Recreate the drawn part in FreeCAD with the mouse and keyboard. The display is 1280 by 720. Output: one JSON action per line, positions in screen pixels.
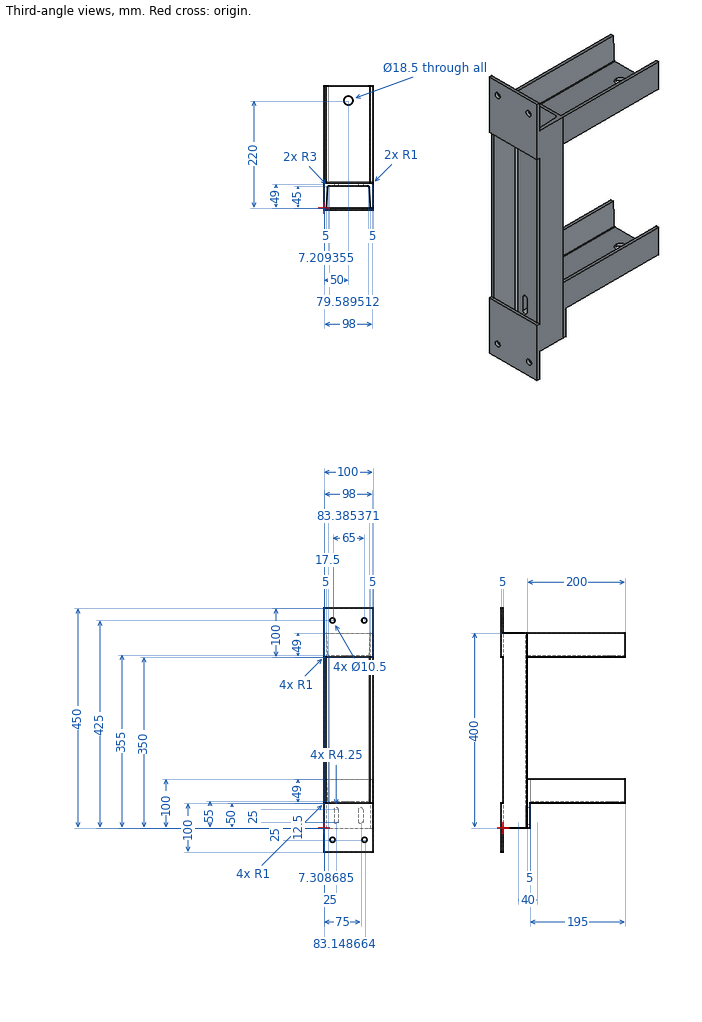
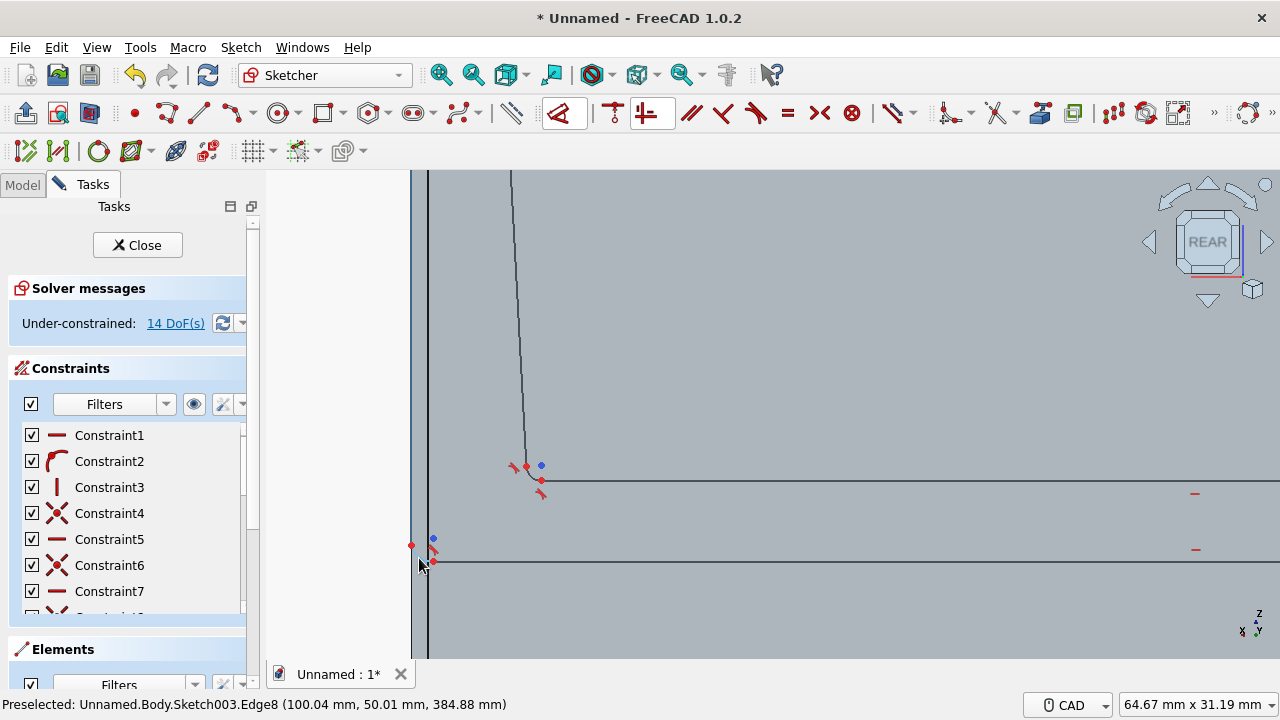
{"action": "left_click", "coordinate": [420, 557]}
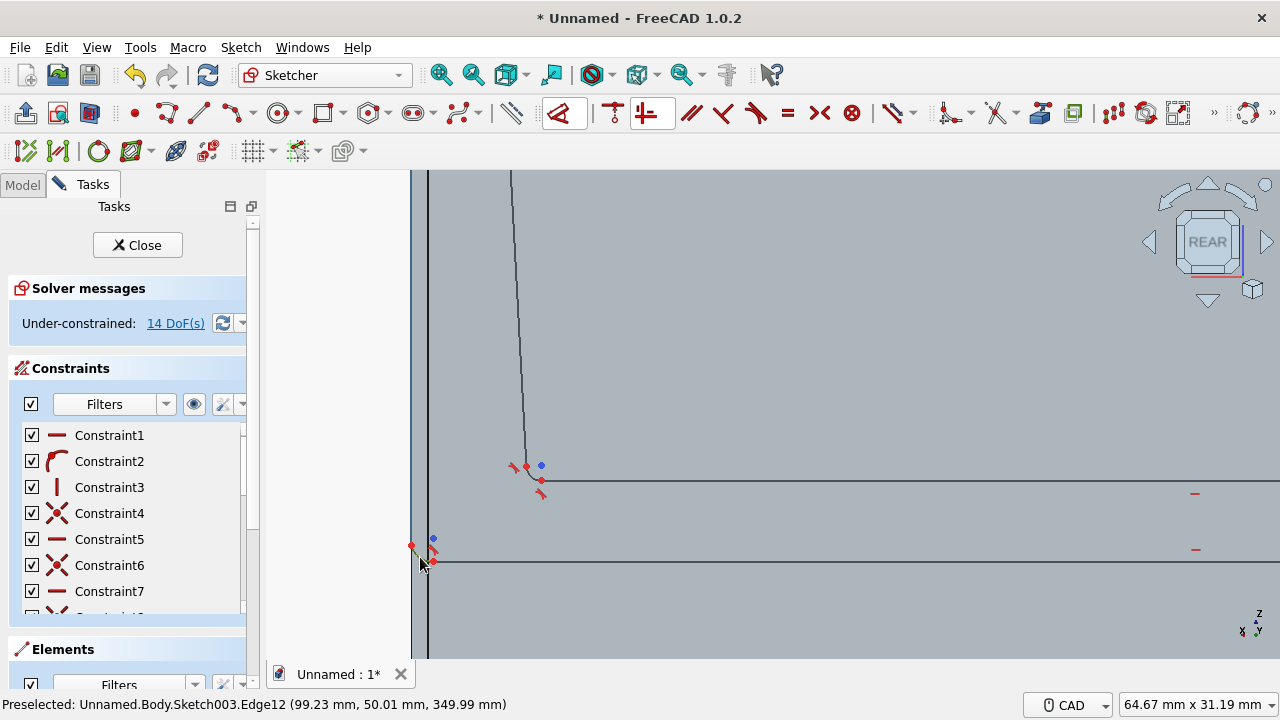
{"action": "left_click", "coordinate": [756, 114]}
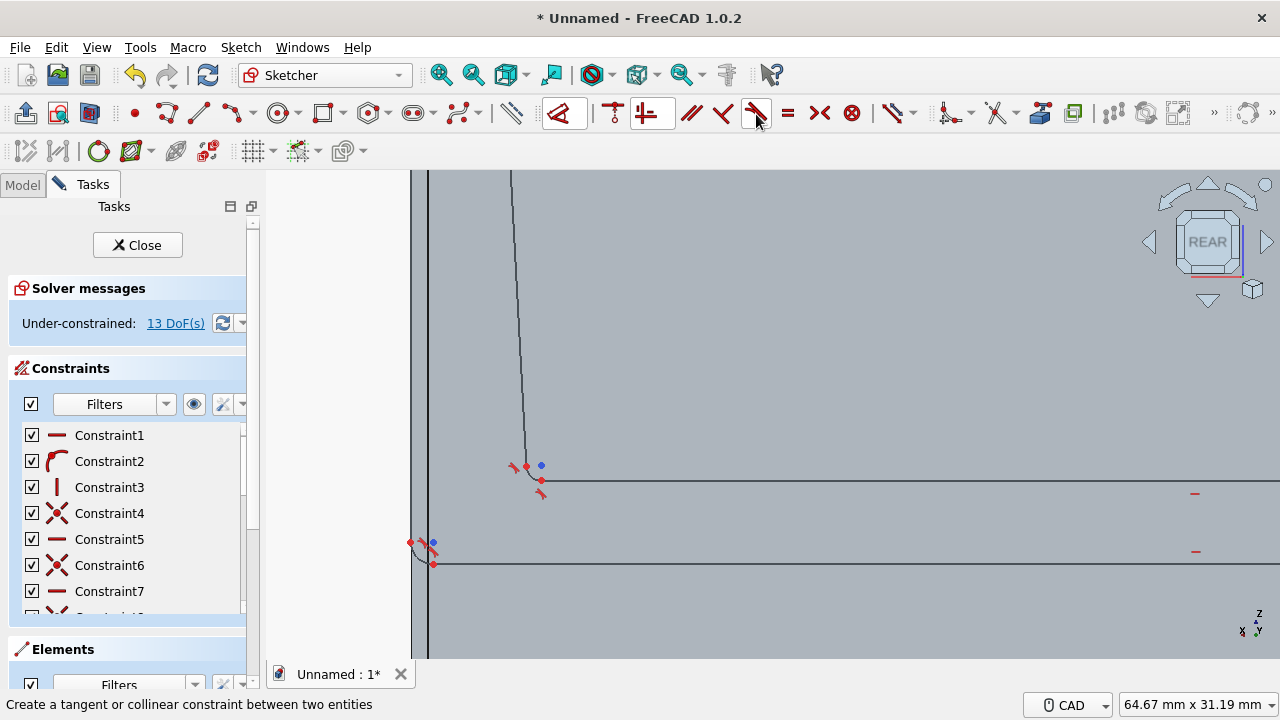
{"action": "scroll", "coordinate": [419, 558], "scroll_direction": "down", "scroll_amount": 5}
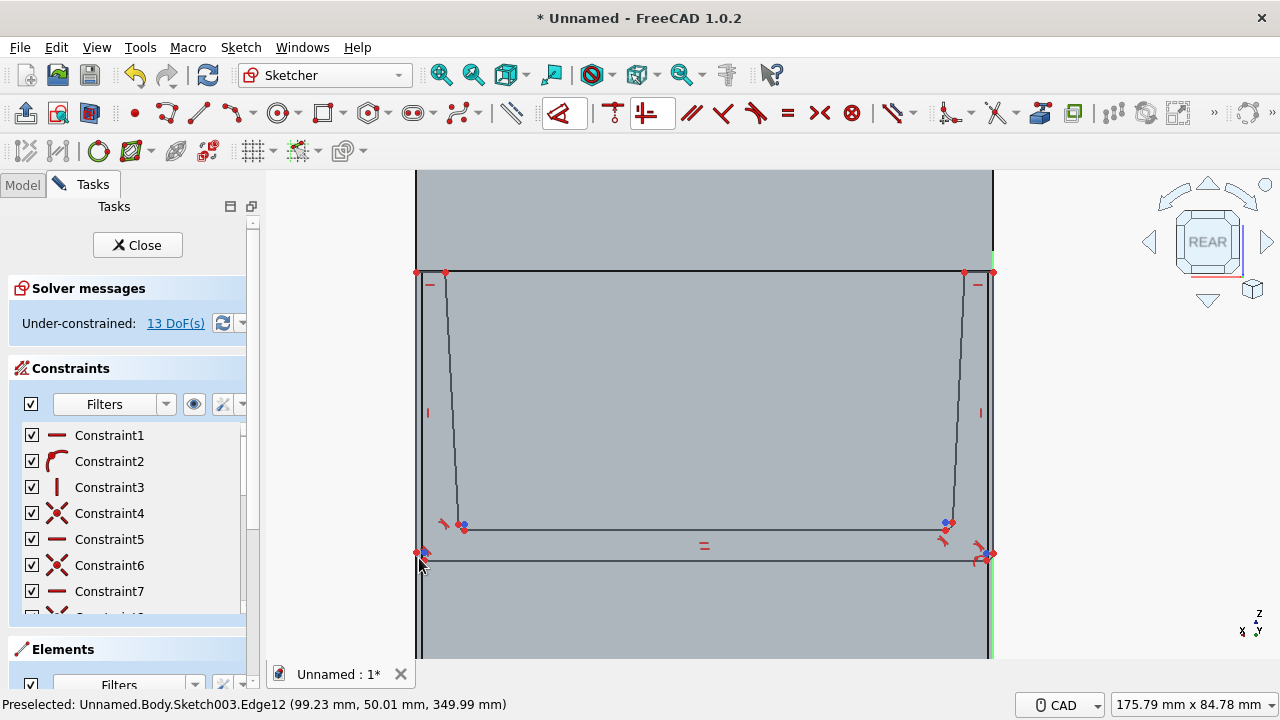
{"action": "scroll", "coordinate": [989, 560], "scroll_direction": "up", "scroll_amount": 8}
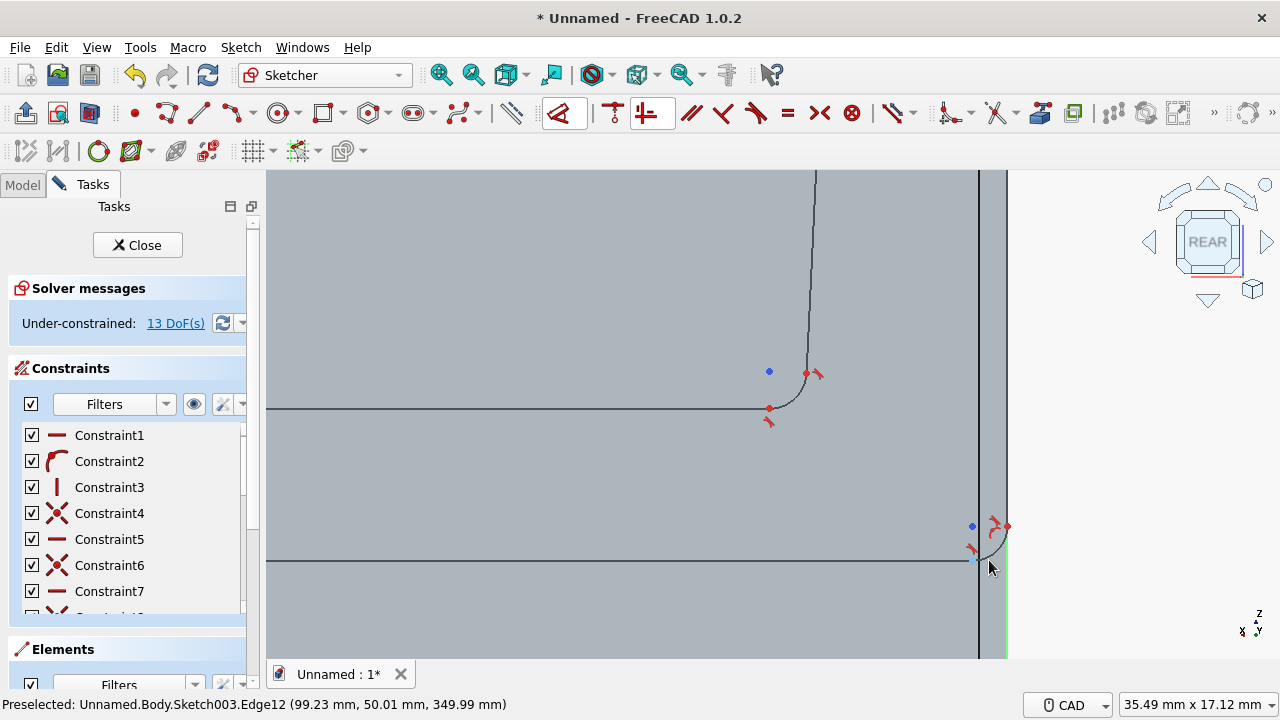
{"action": "left_click", "coordinate": [989, 557]}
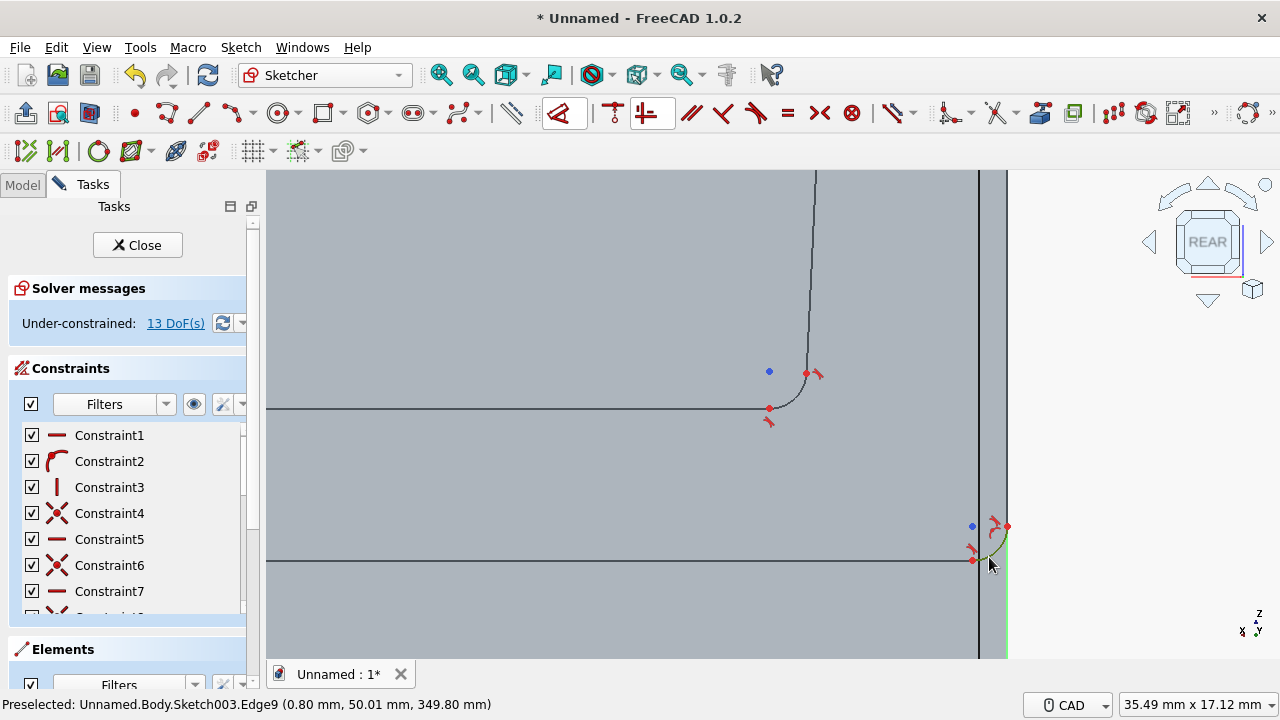
{"action": "left_click", "coordinate": [786, 405]}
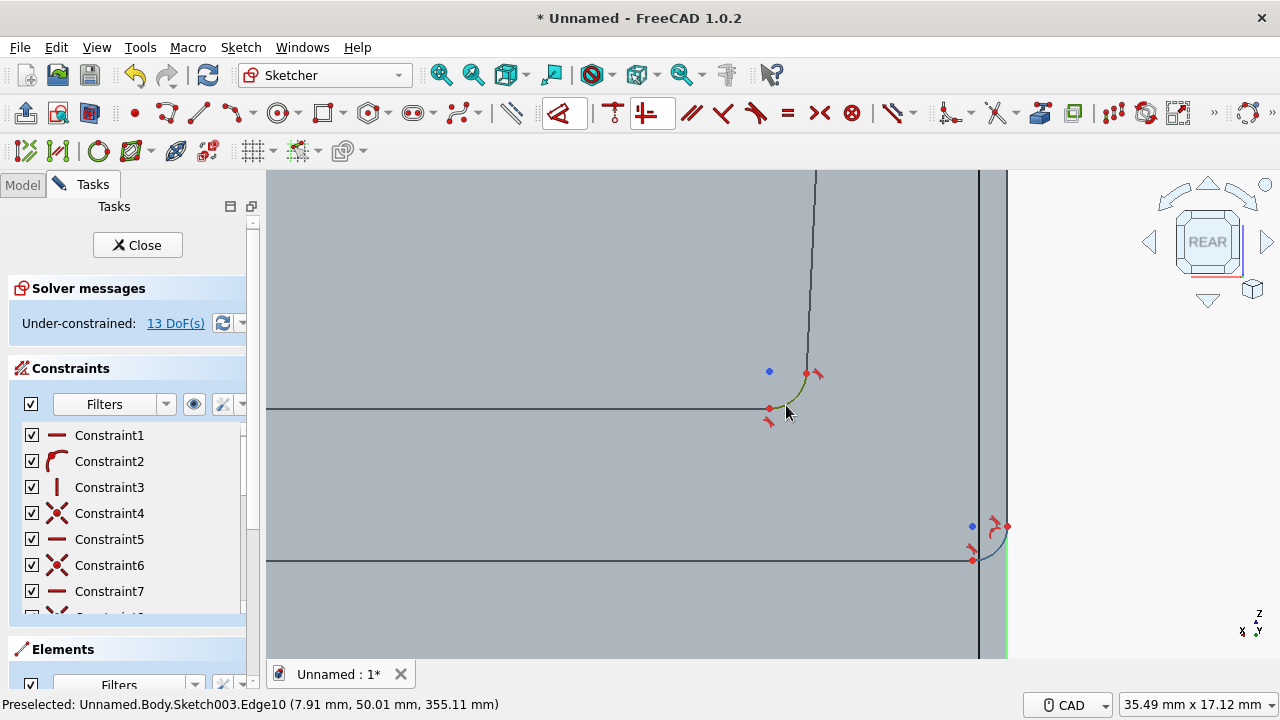
{"action": "scroll", "coordinate": [989, 560], "scroll_direction": "down", "scroll_amount": 8}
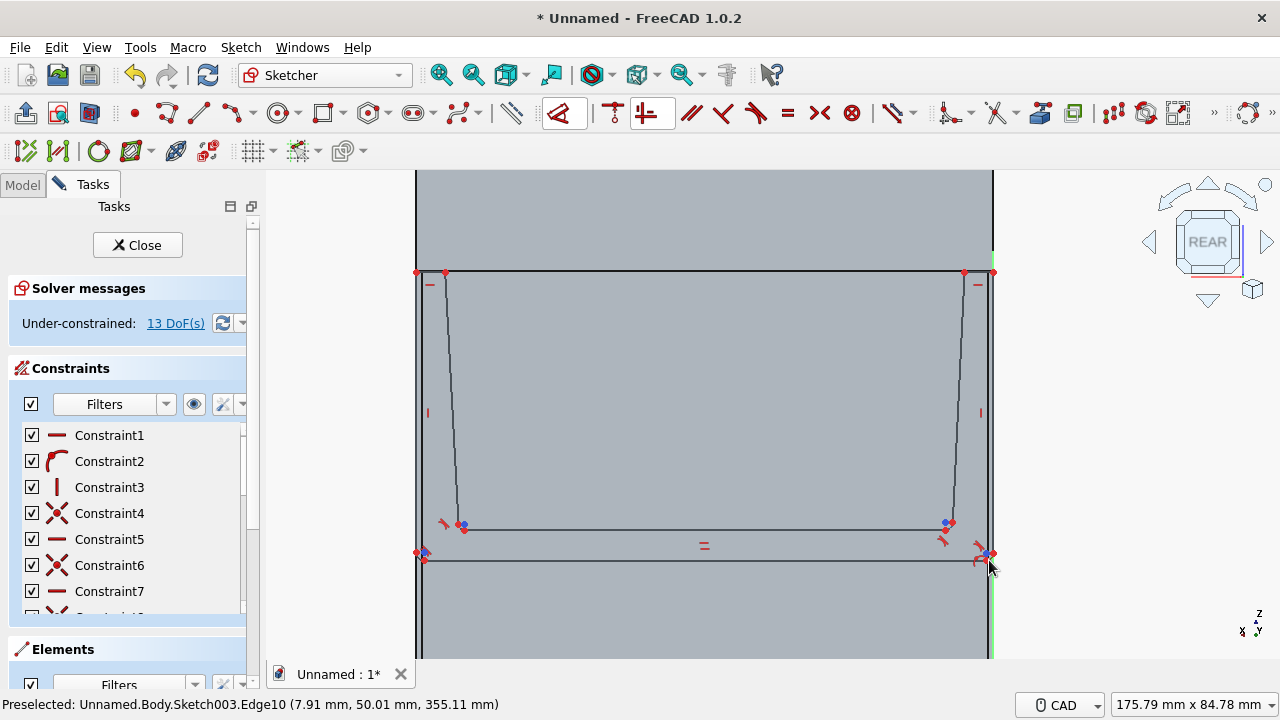
{"action": "scroll", "coordinate": [459, 527], "scroll_direction": "up", "scroll_amount": 9}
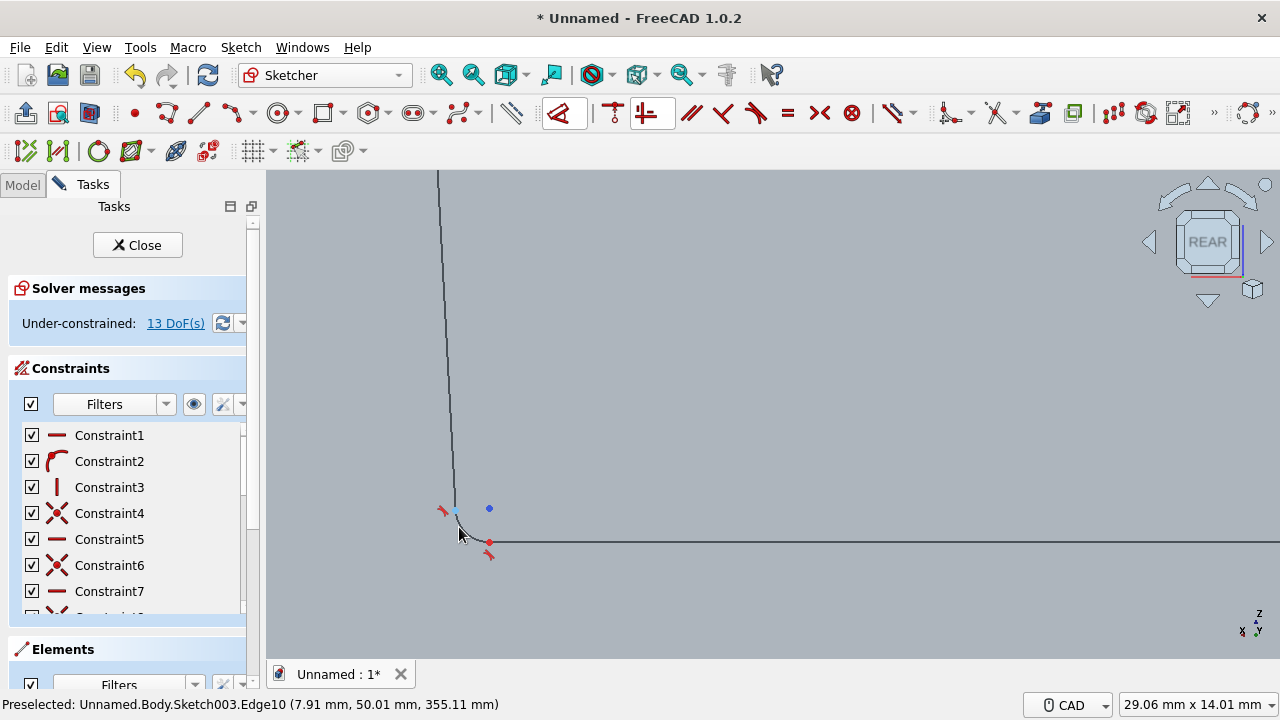
{"action": "left_click", "coordinate": [460, 525]}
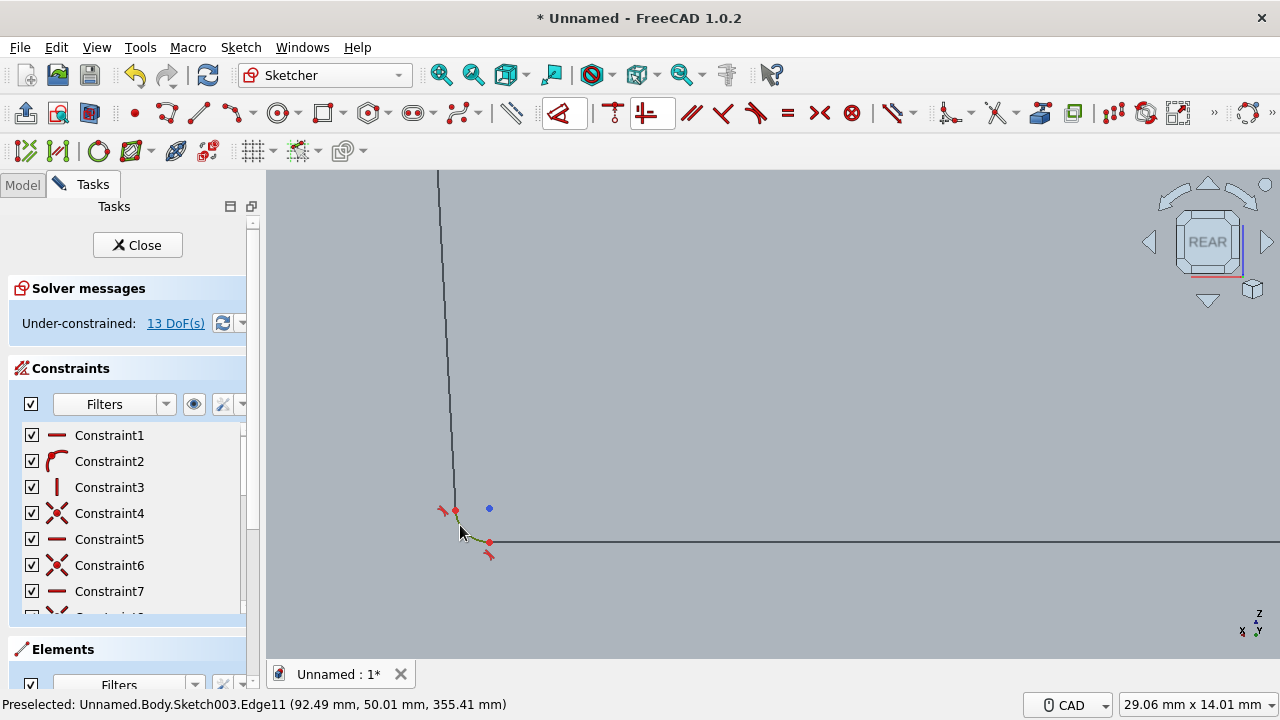
{"action": "scroll", "coordinate": [459, 527], "scroll_direction": "down", "scroll_amount": 9}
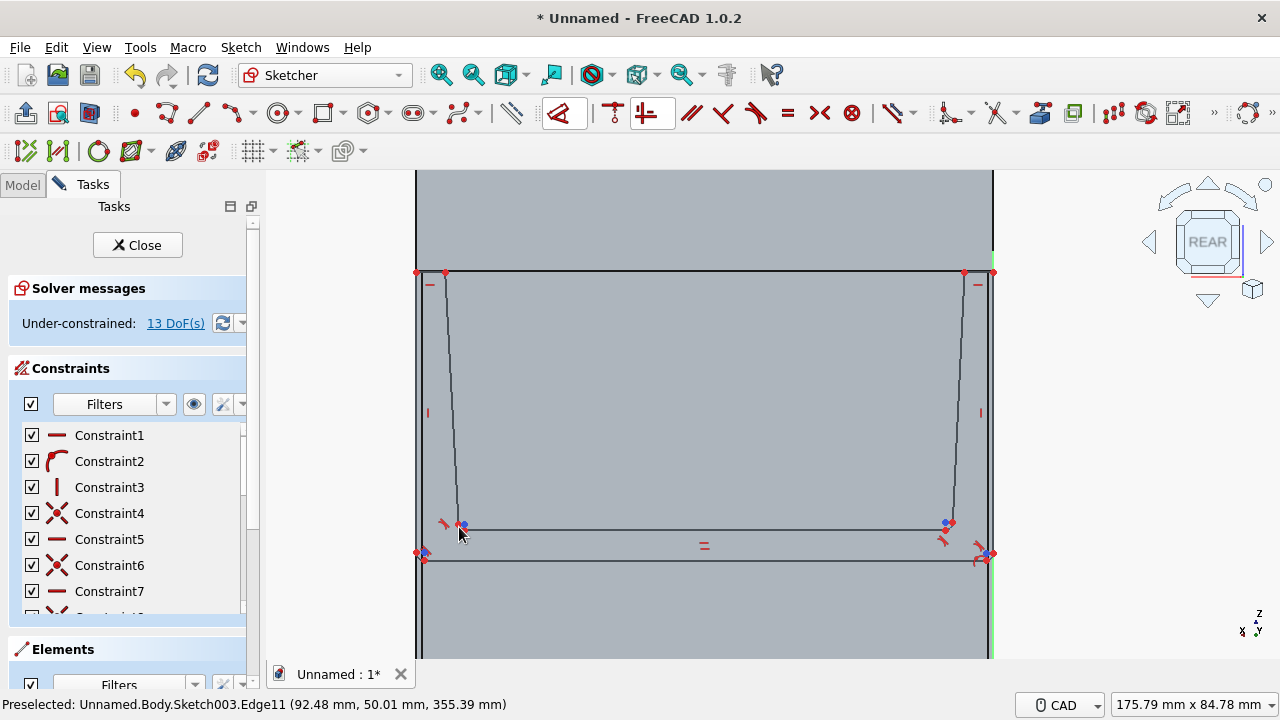
{"action": "scroll", "coordinate": [417, 556], "scroll_direction": "up", "scroll_amount": 7}